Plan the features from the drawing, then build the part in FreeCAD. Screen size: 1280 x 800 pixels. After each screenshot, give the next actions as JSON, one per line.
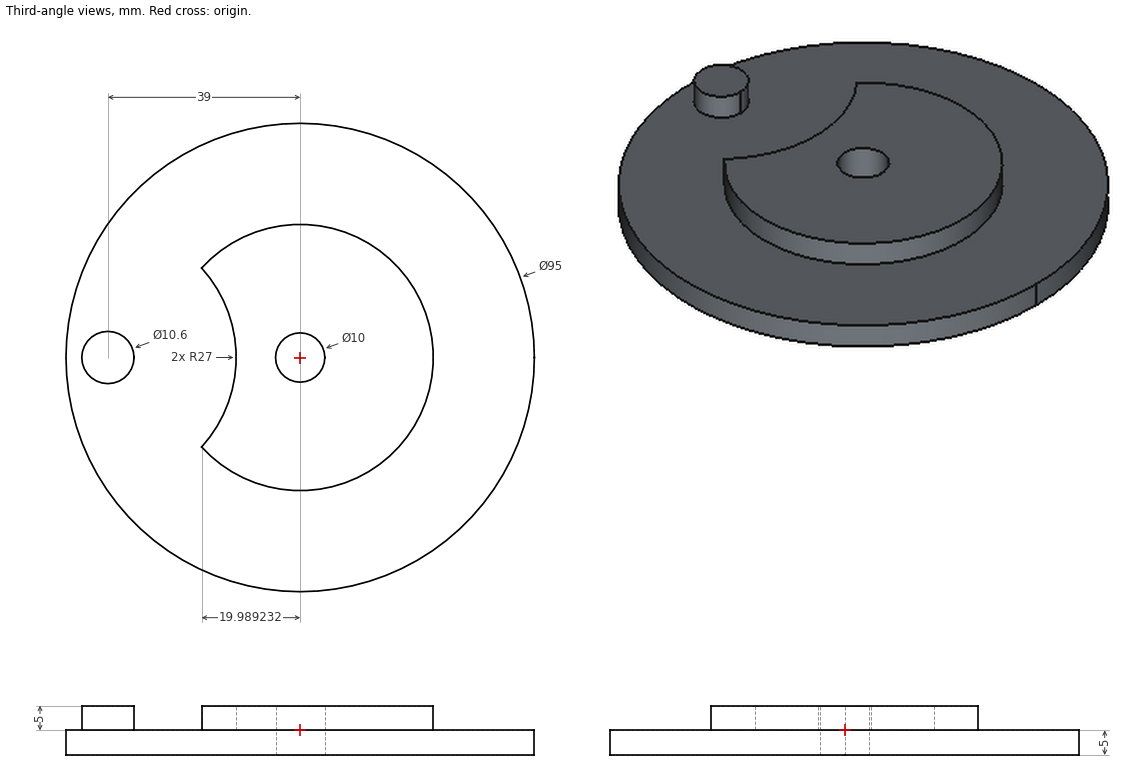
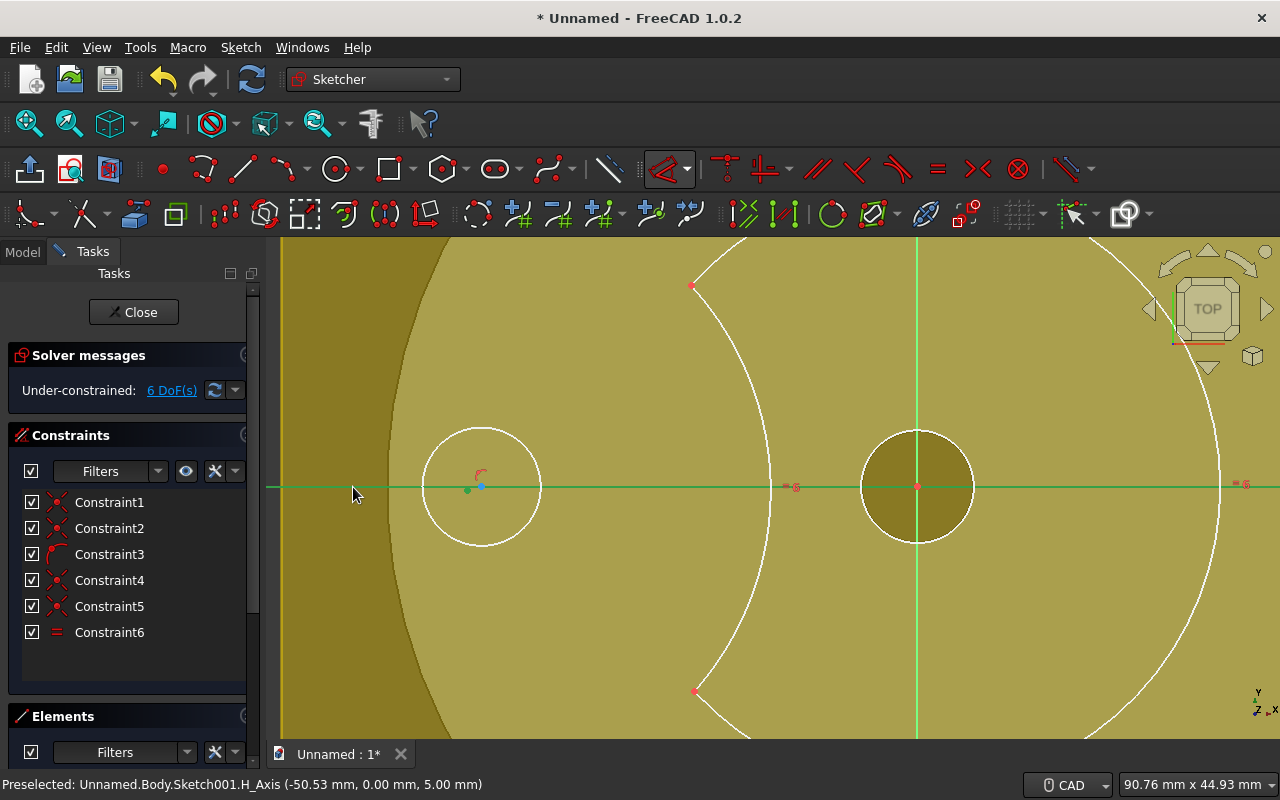
{"action": "key", "text": "c"}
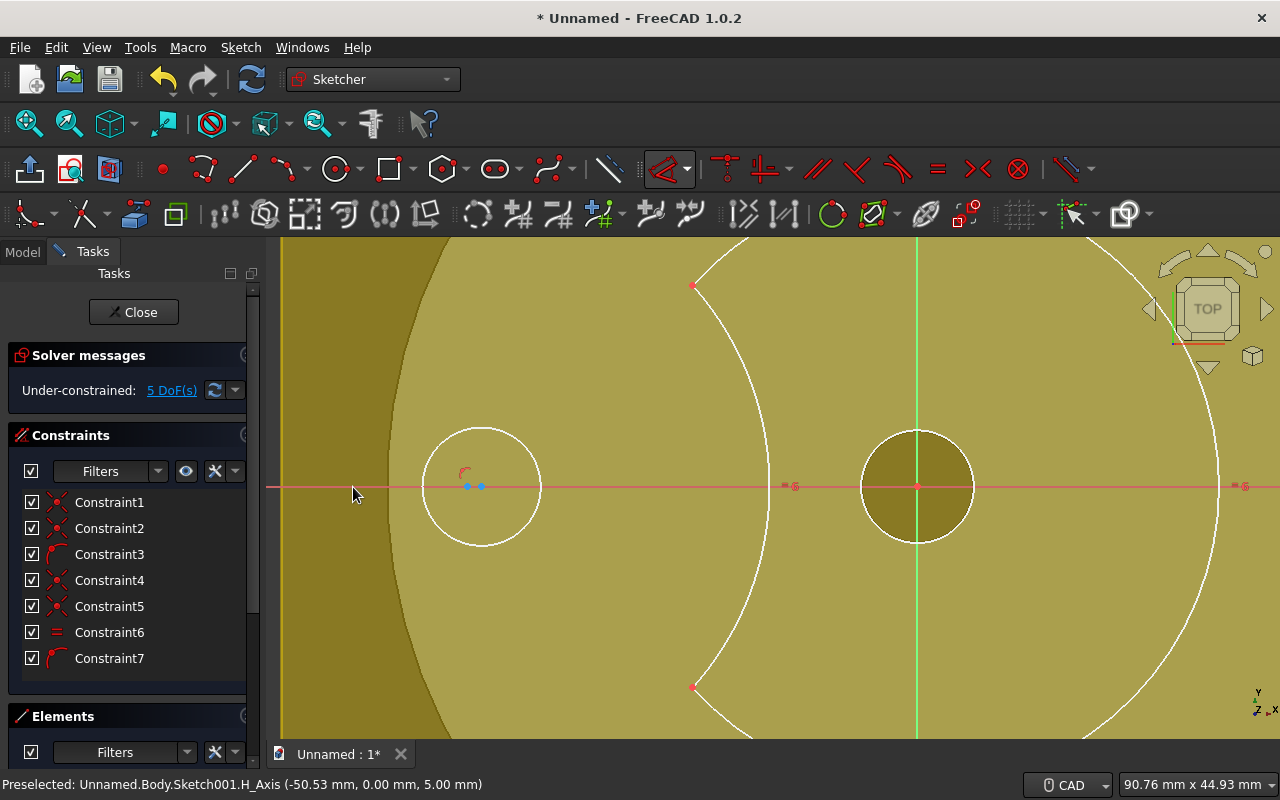
{"action": "left_click", "coordinate": [757, 574]}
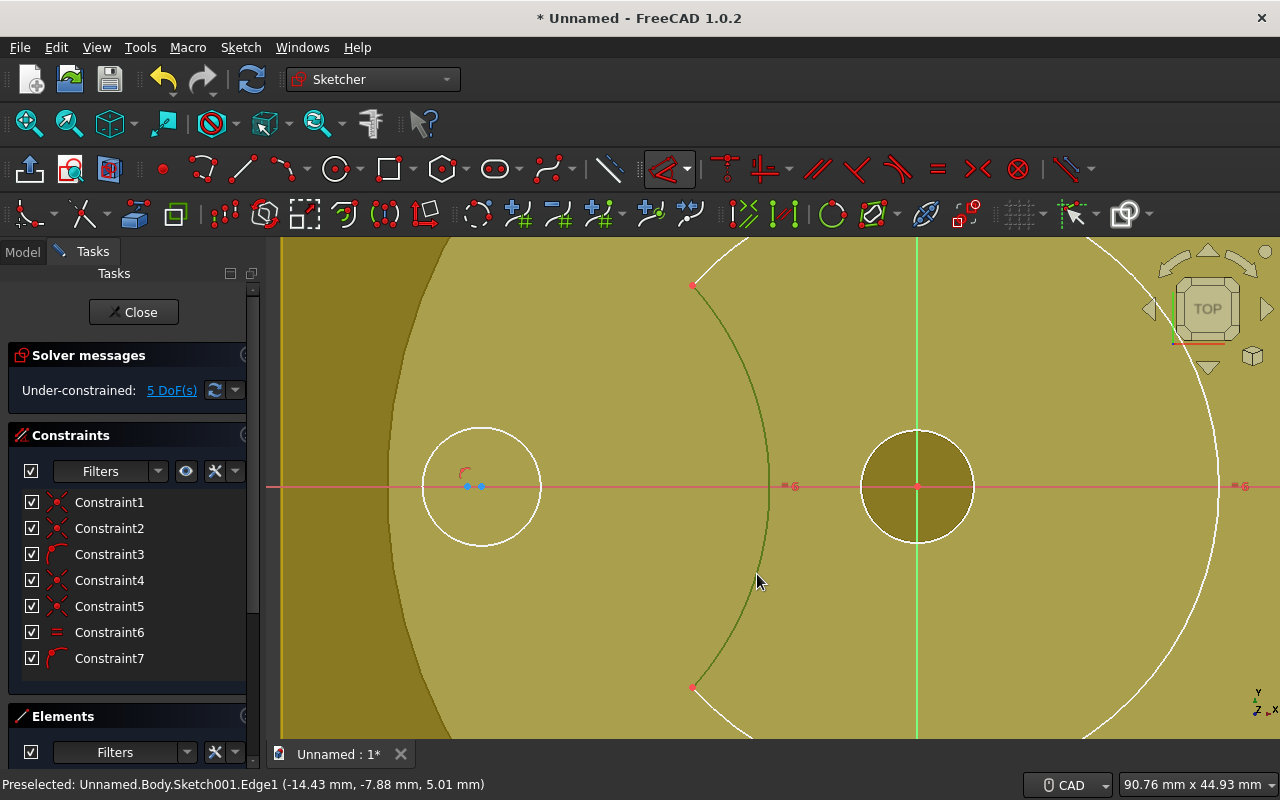
{"action": "key", "text": "k r"}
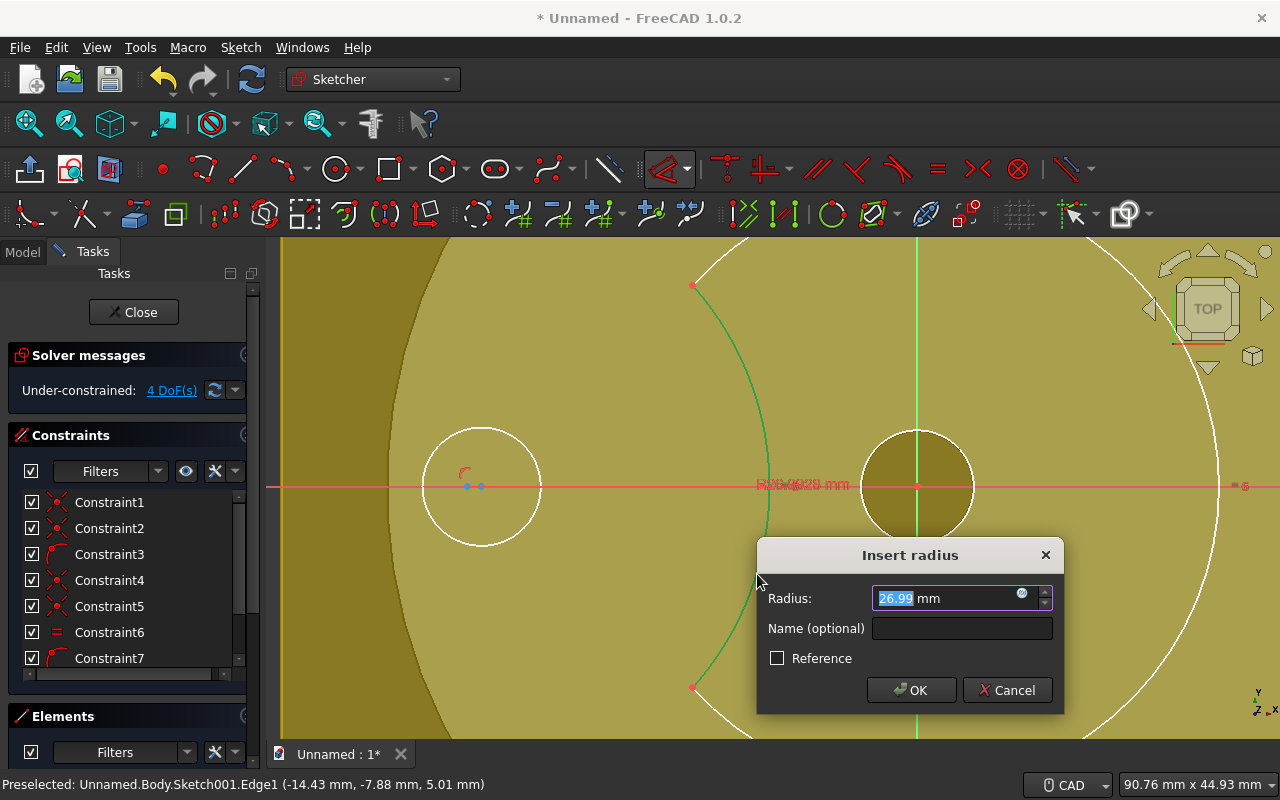
{"action": "type", "text": "27"}
{"action": "key", "text": "Return"}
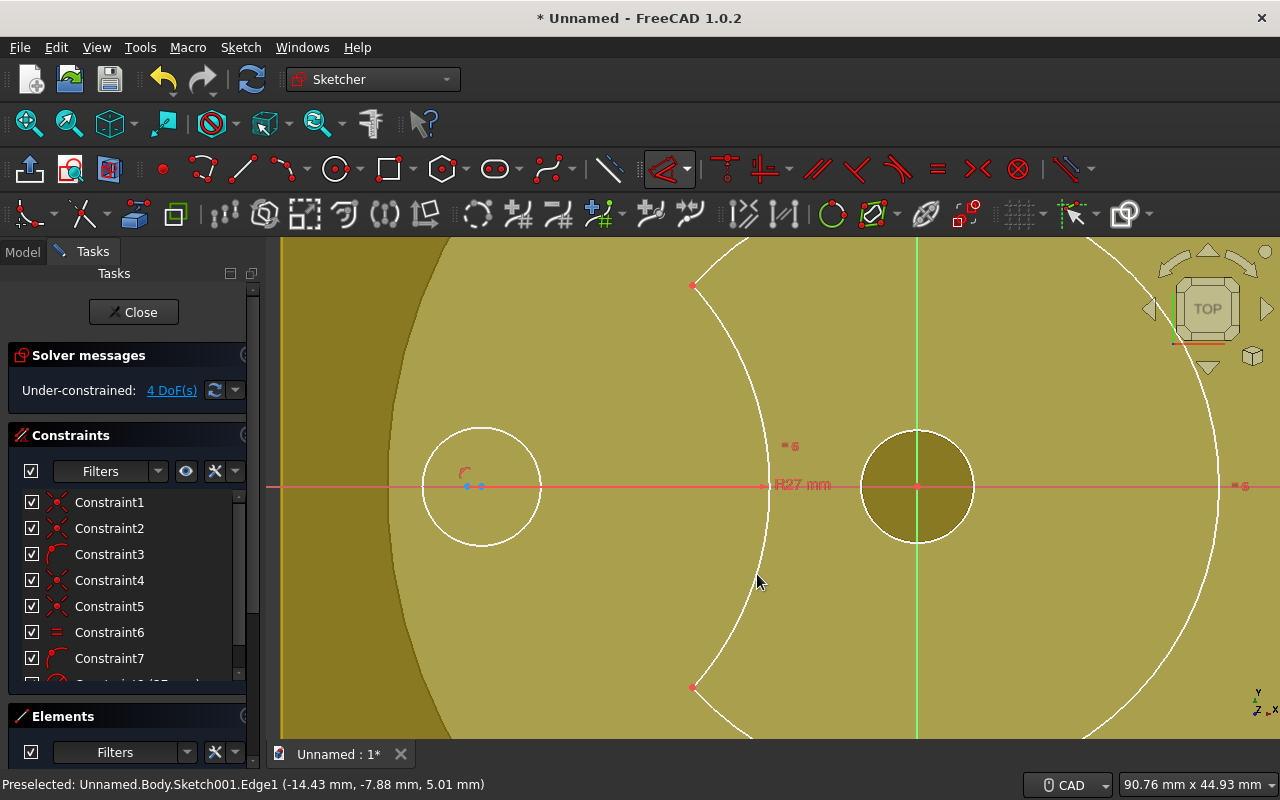
{"action": "left_click", "coordinate": [523, 445]}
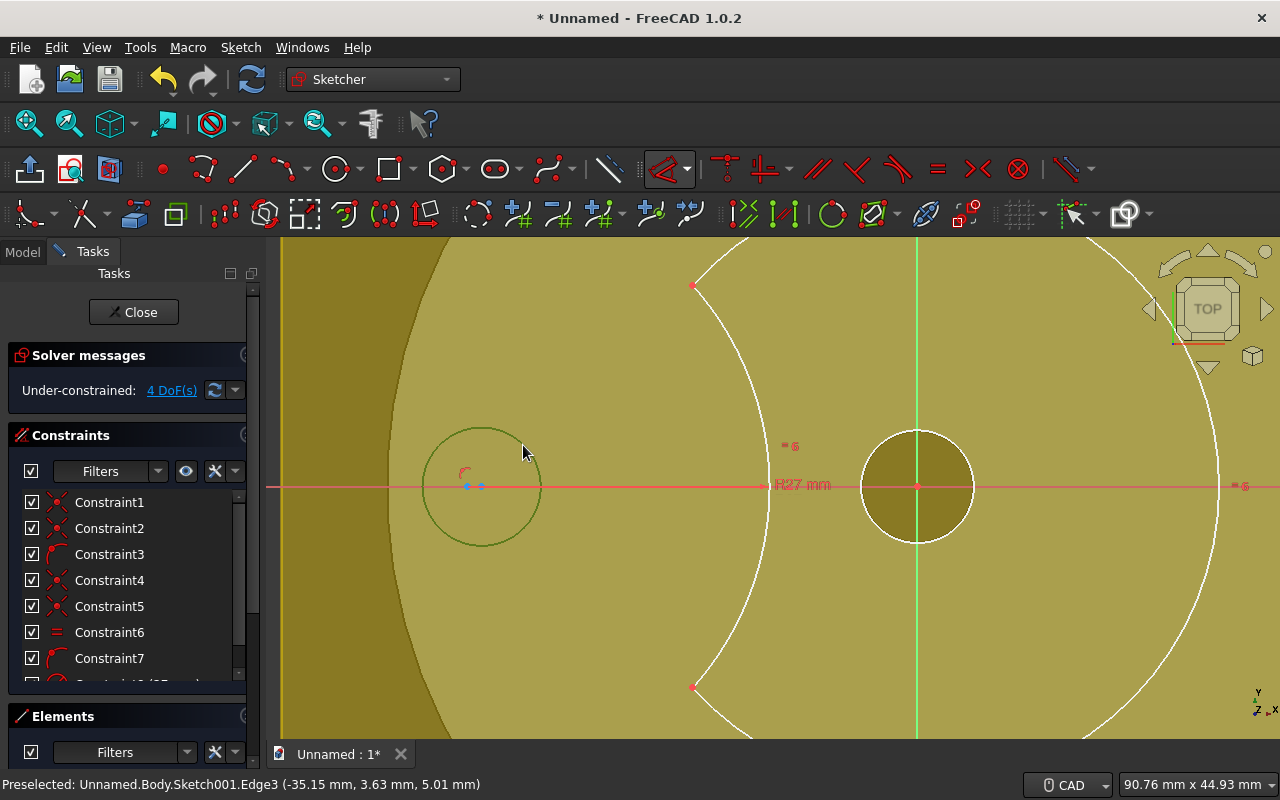
{"action": "key", "text": "k o"}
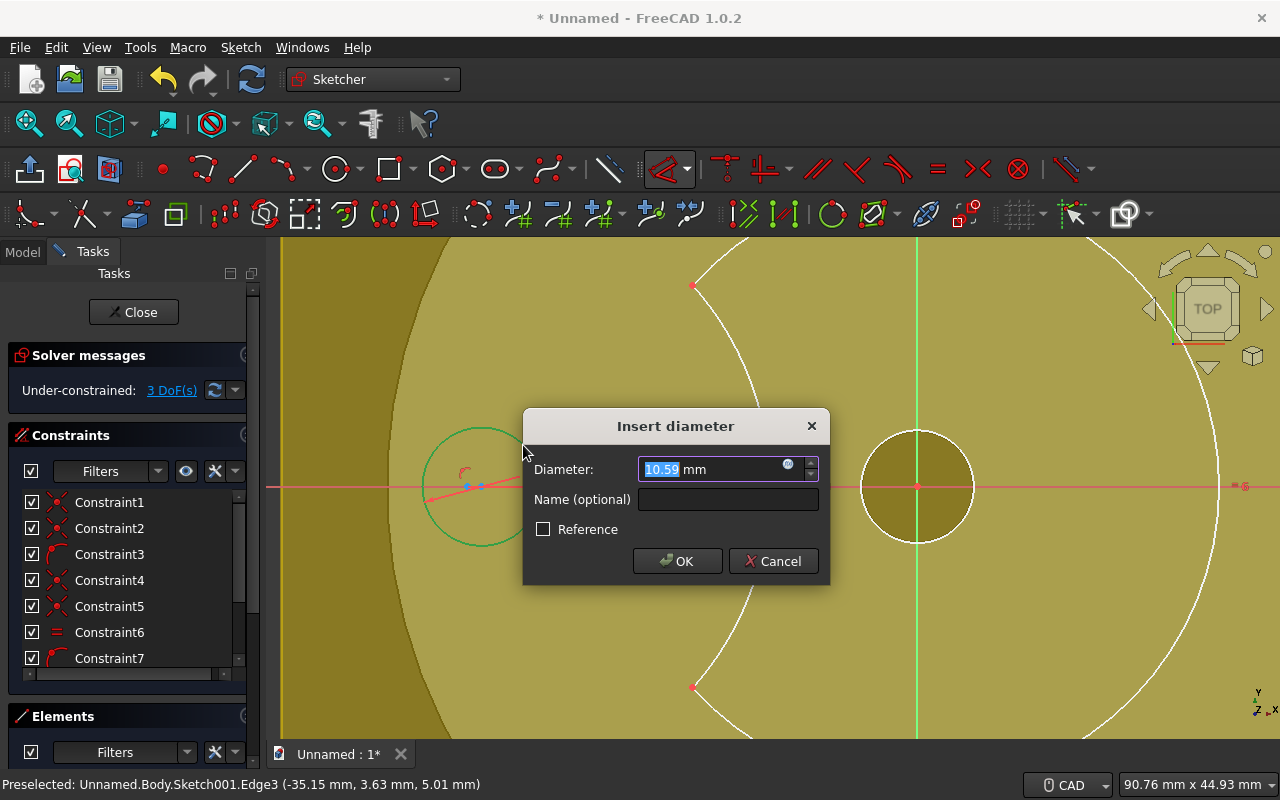
{"action": "type", "text": "10.6"}
{"action": "key", "text": "Return"}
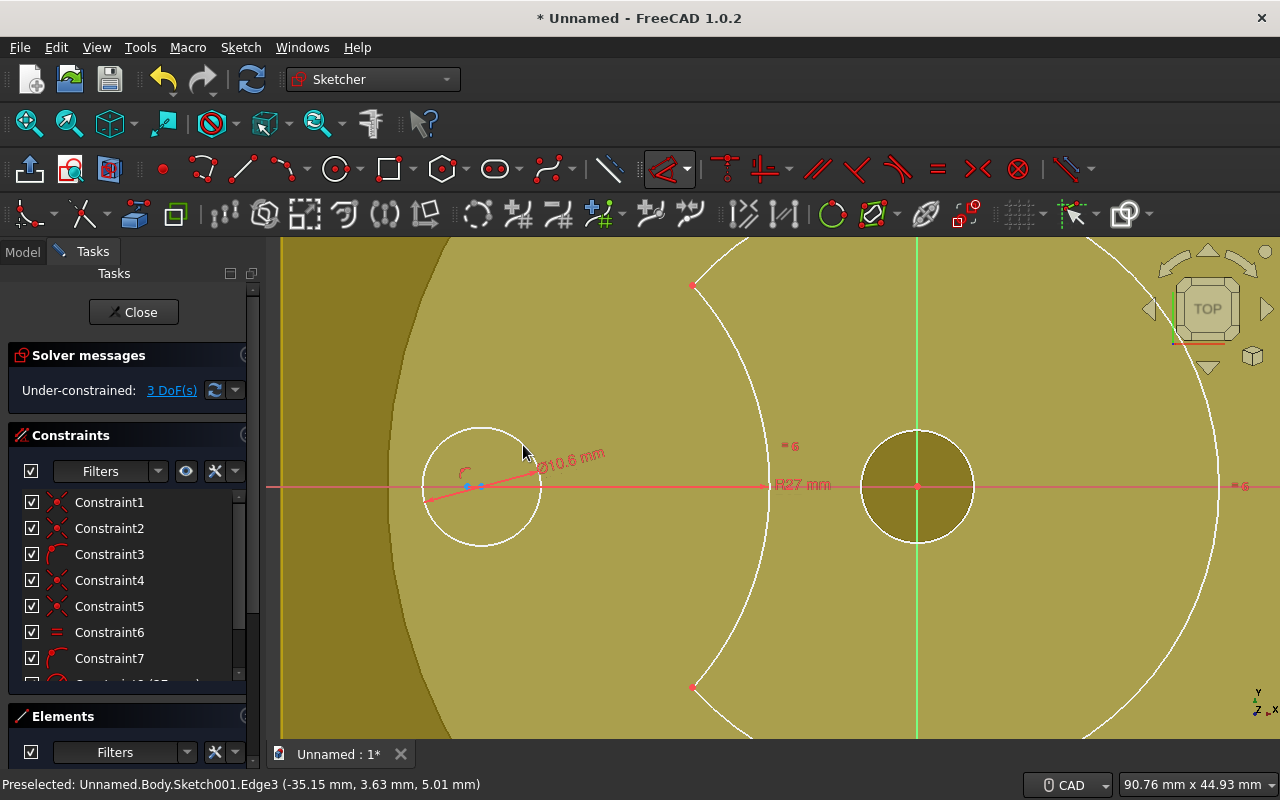
{"action": "left_click", "coordinate": [957, 447]}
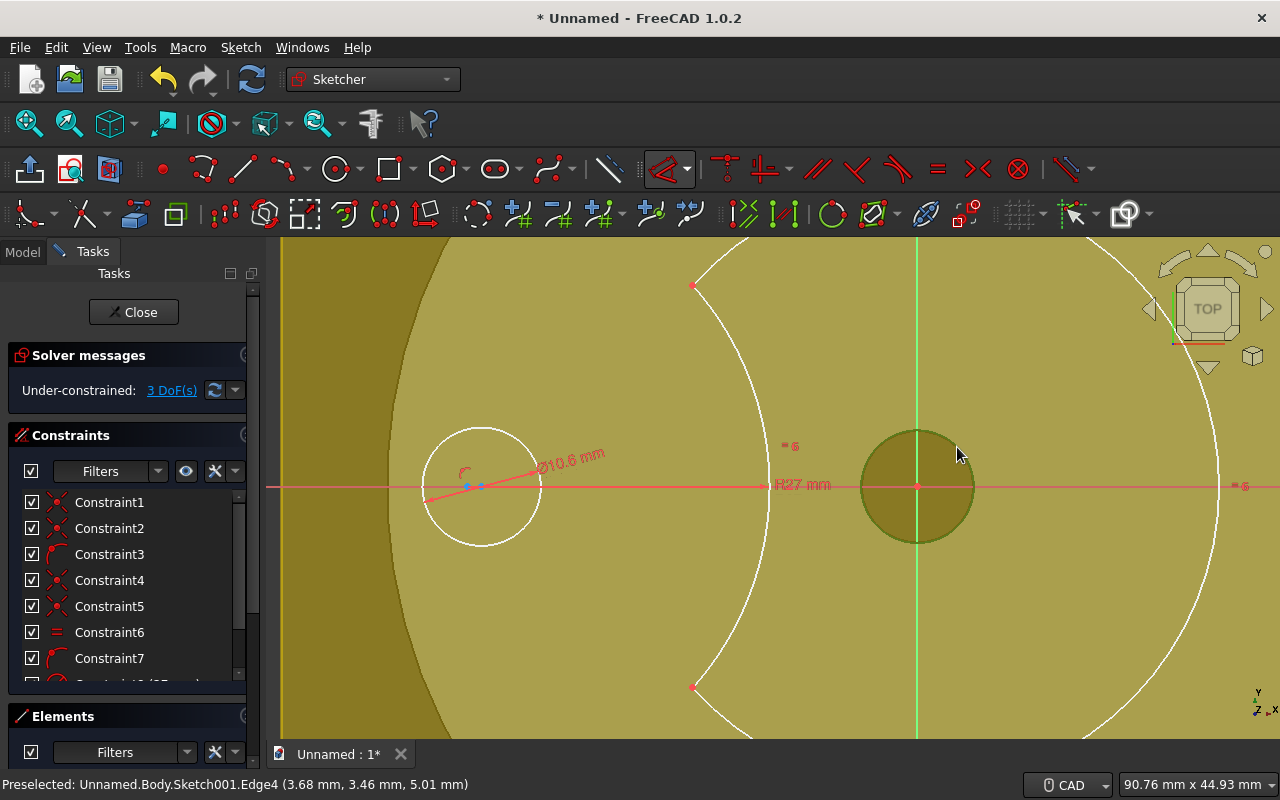
{"action": "key", "text": "k o"}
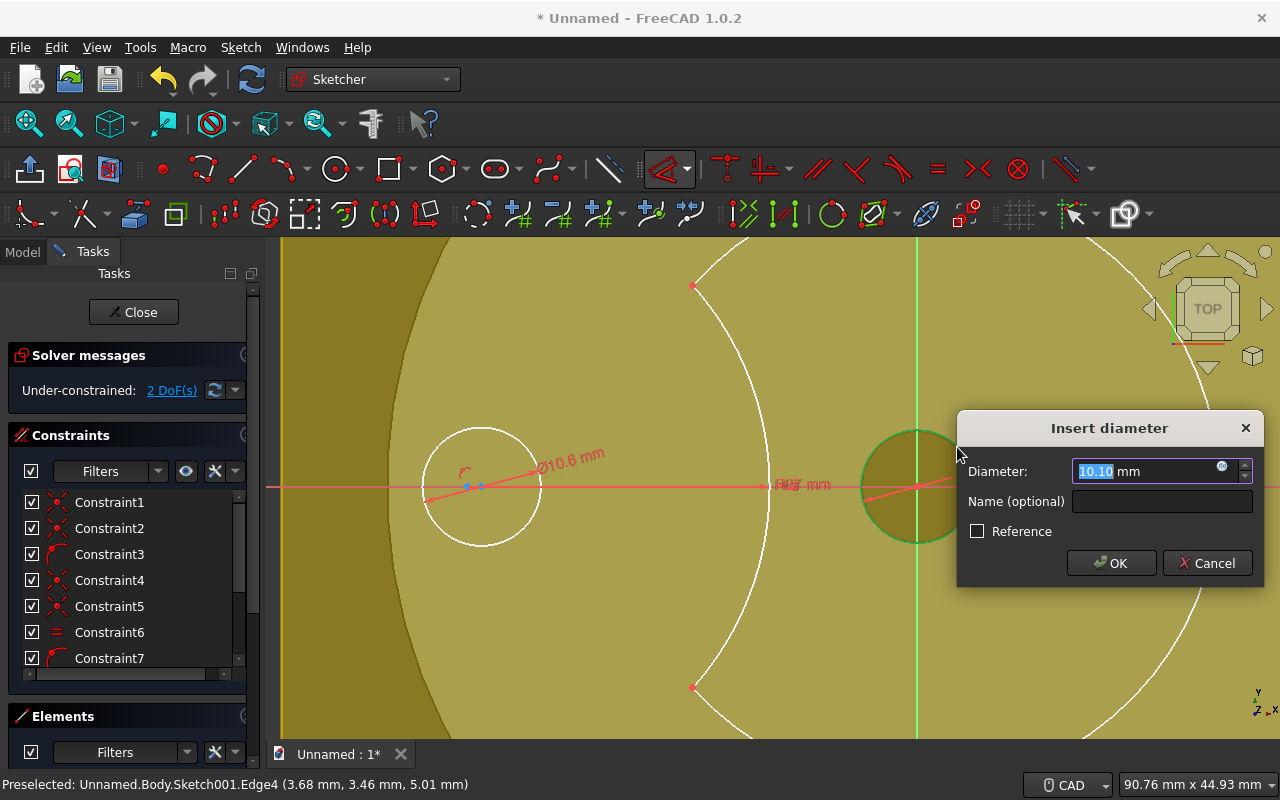
{"action": "type", "text": "10"}
{"action": "key", "text": "Return"}